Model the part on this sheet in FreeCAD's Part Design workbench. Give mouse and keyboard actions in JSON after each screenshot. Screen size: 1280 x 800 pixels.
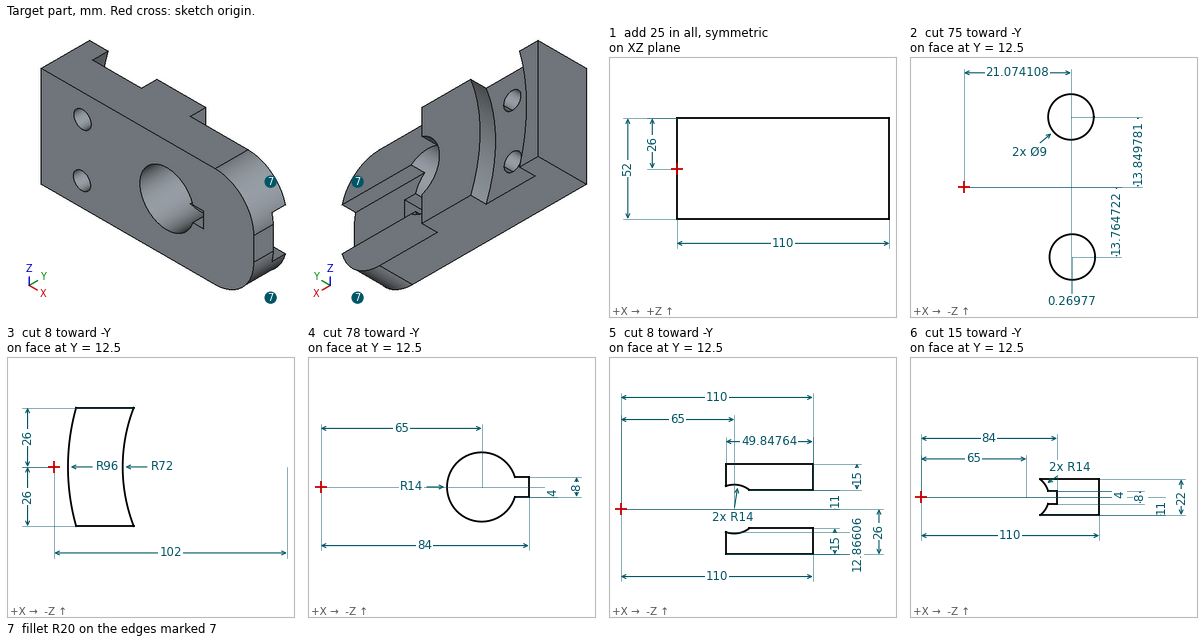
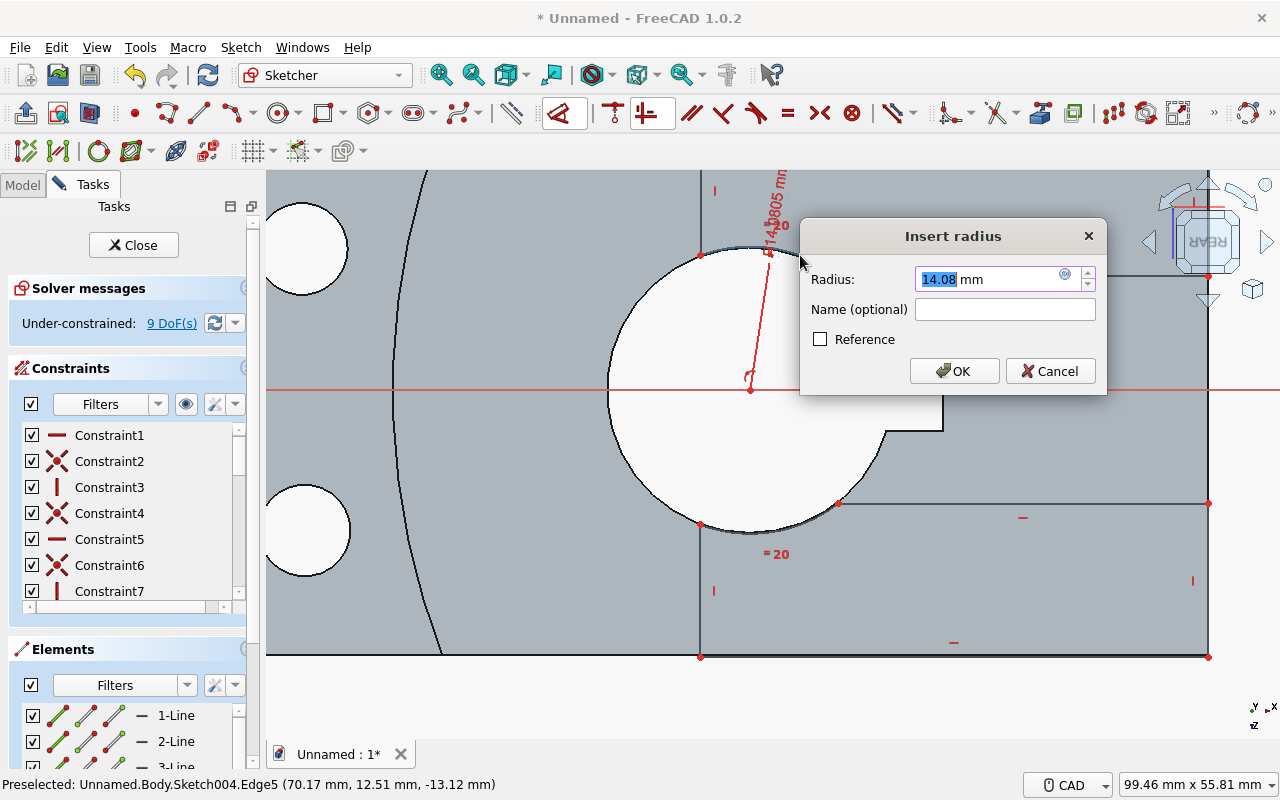
{"action": "type", "text": "14"}
{"action": "key", "text": "Return"}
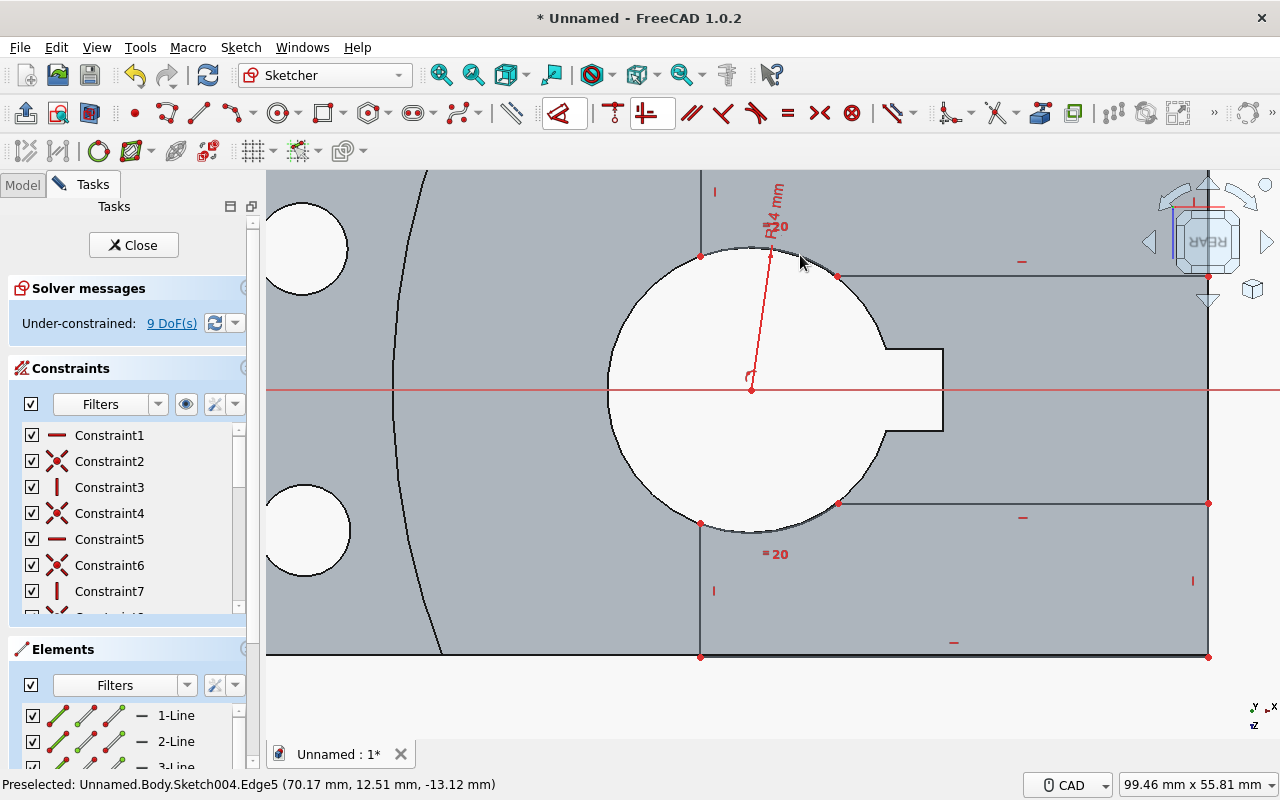
{"action": "scroll", "coordinate": [774, 533], "scroll_direction": "down", "scroll_amount": 3}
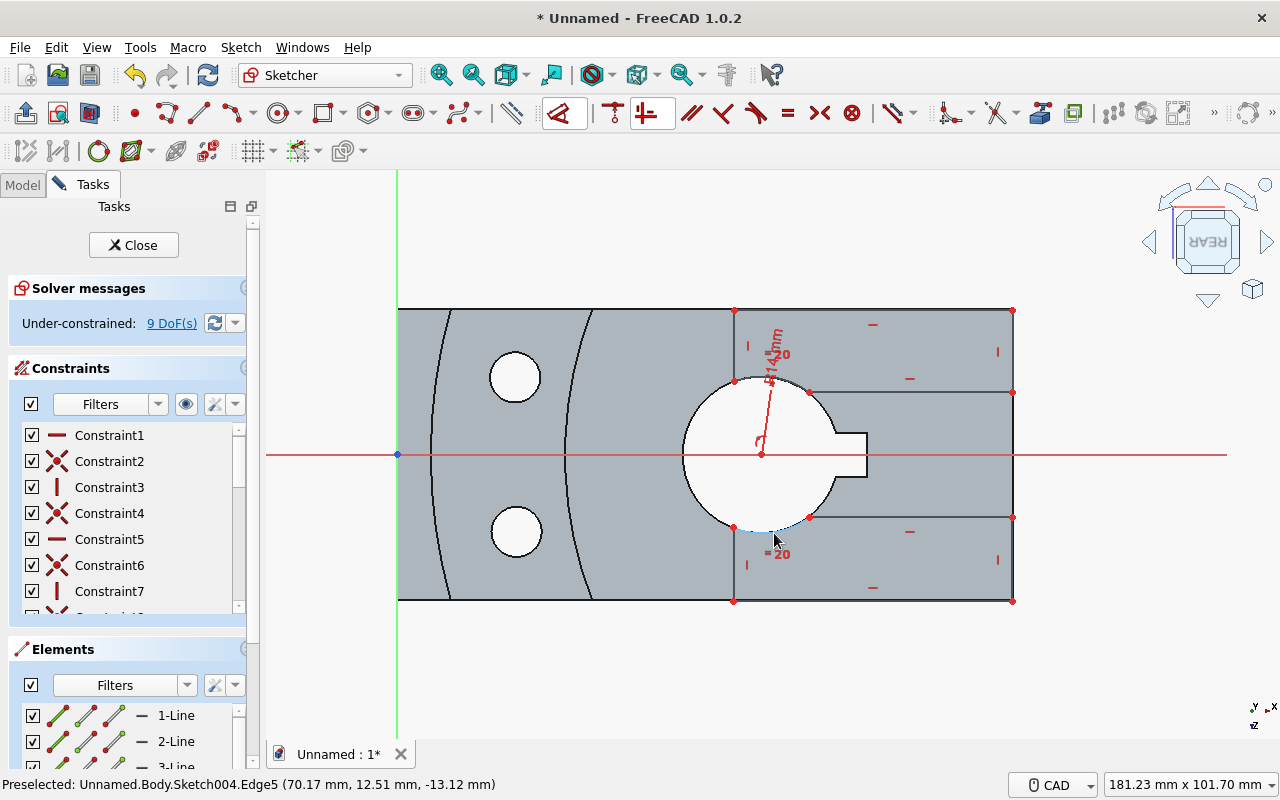
{"action": "left_click", "coordinate": [1013, 368]}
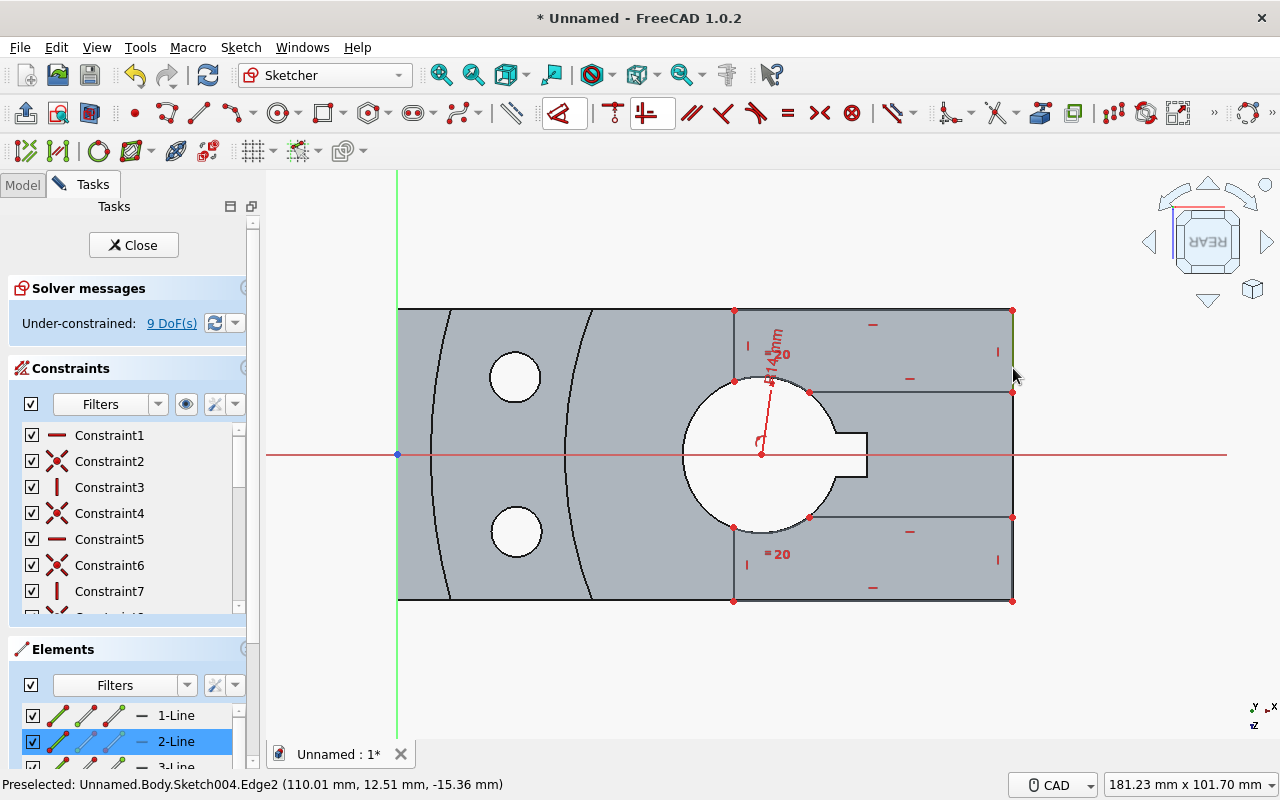
{"action": "key", "text": "i"}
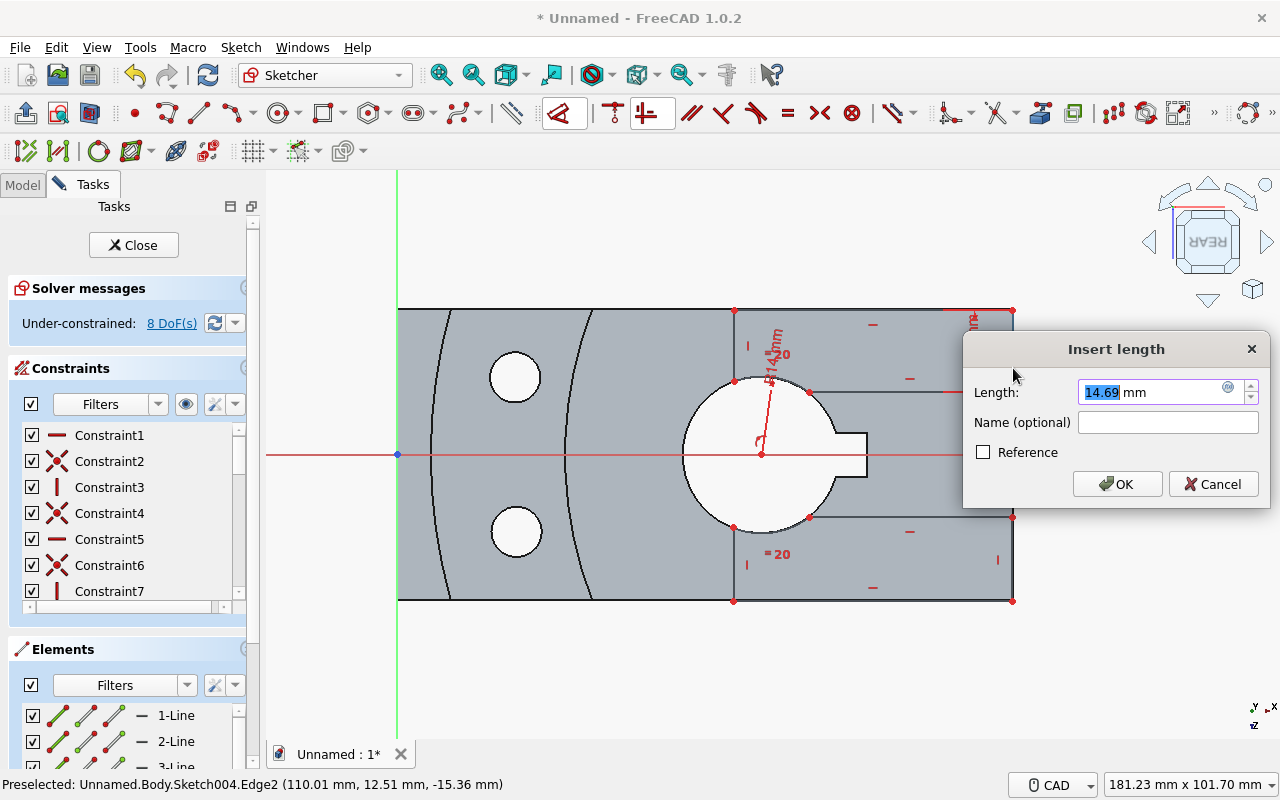
{"action": "type", "text": "15"}
{"action": "key", "text": "Return"}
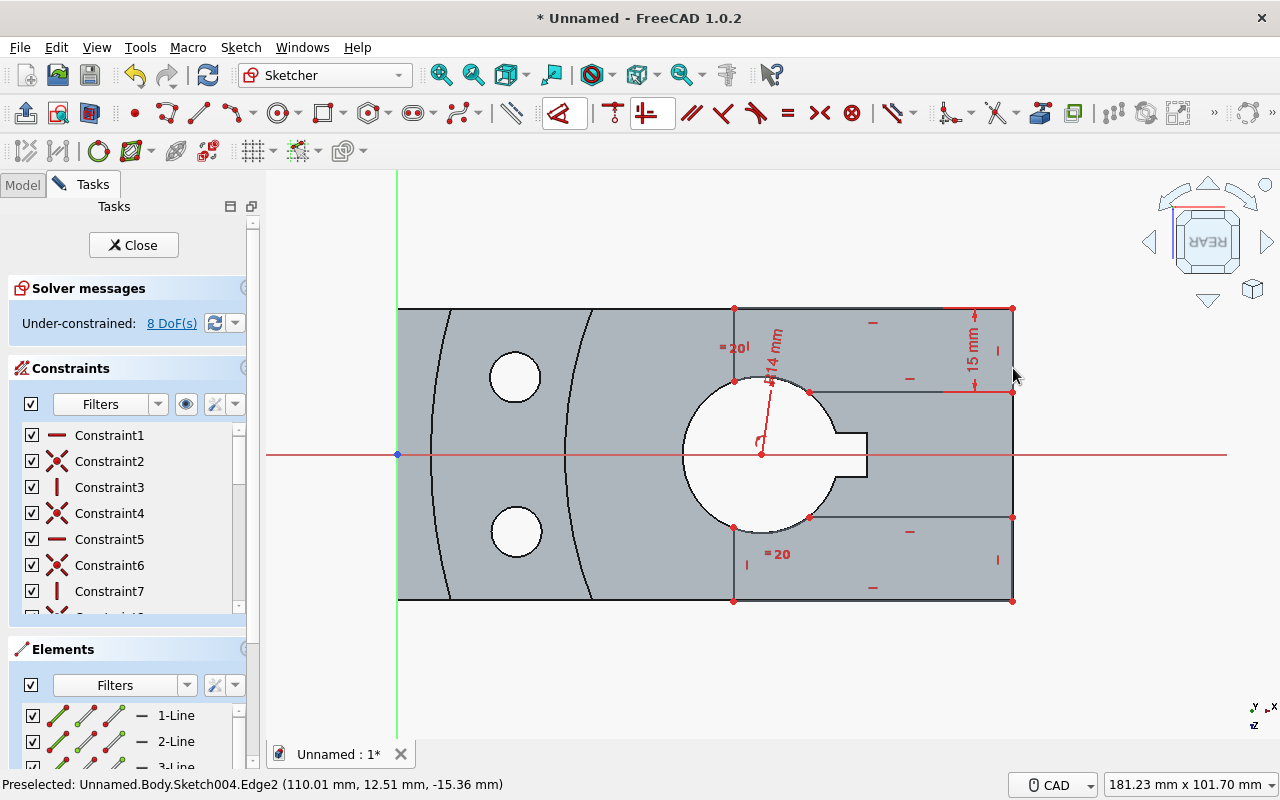
{"action": "left_click", "coordinate": [1012, 576]}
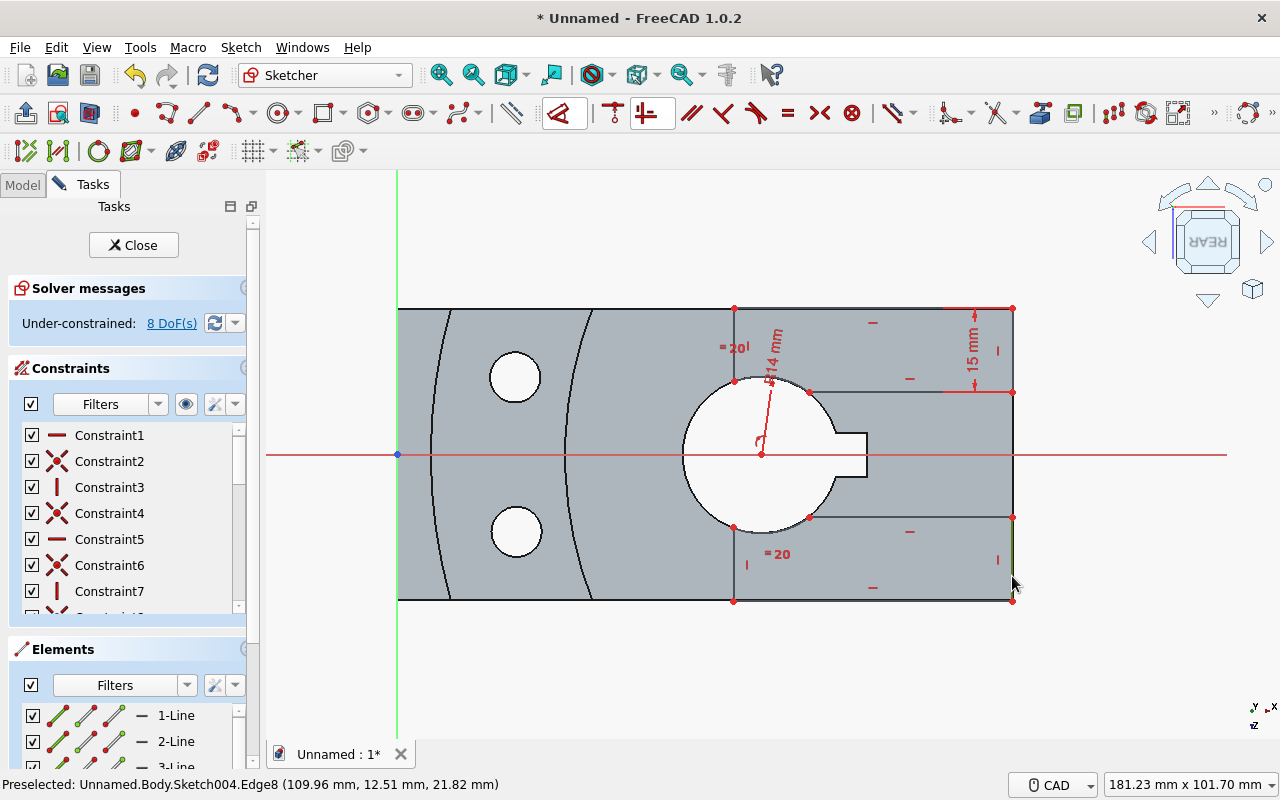
{"action": "left_click", "coordinate": [582, 114]}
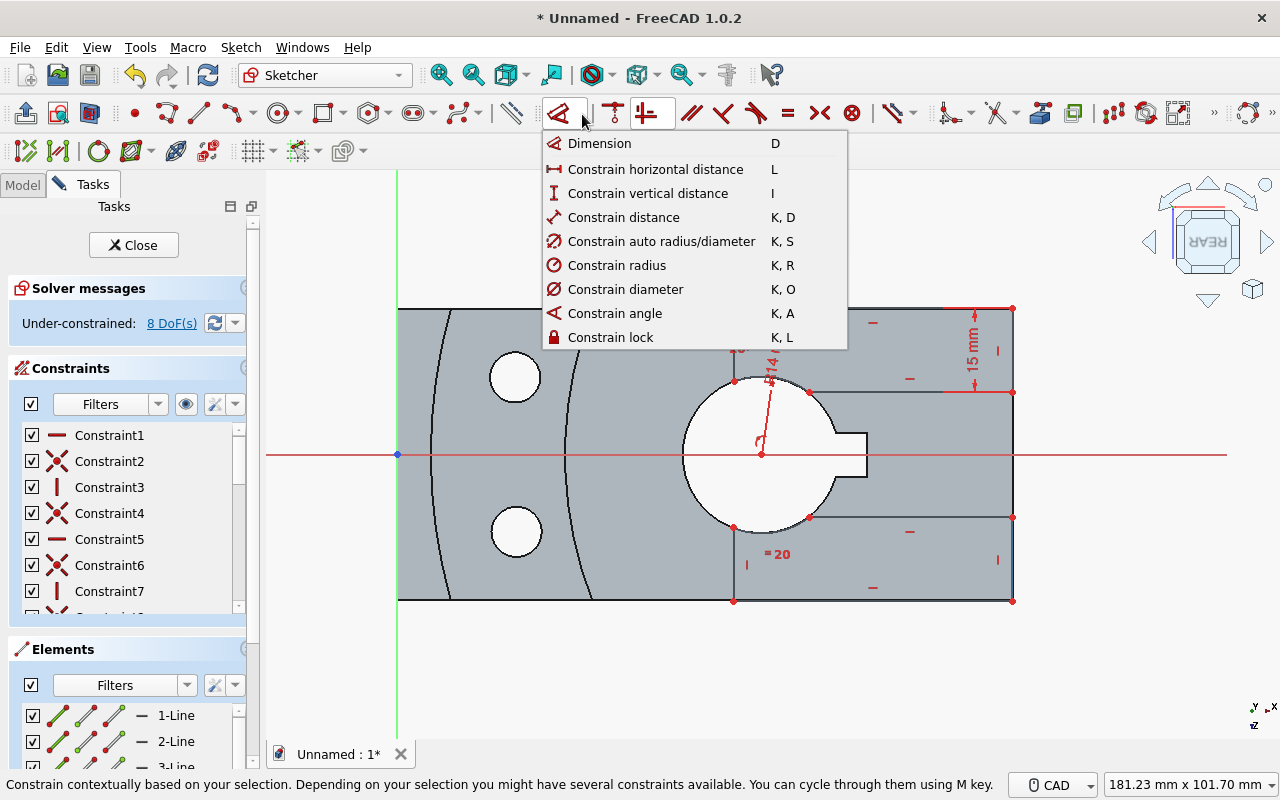
{"action": "left_click", "coordinate": [695, 193]}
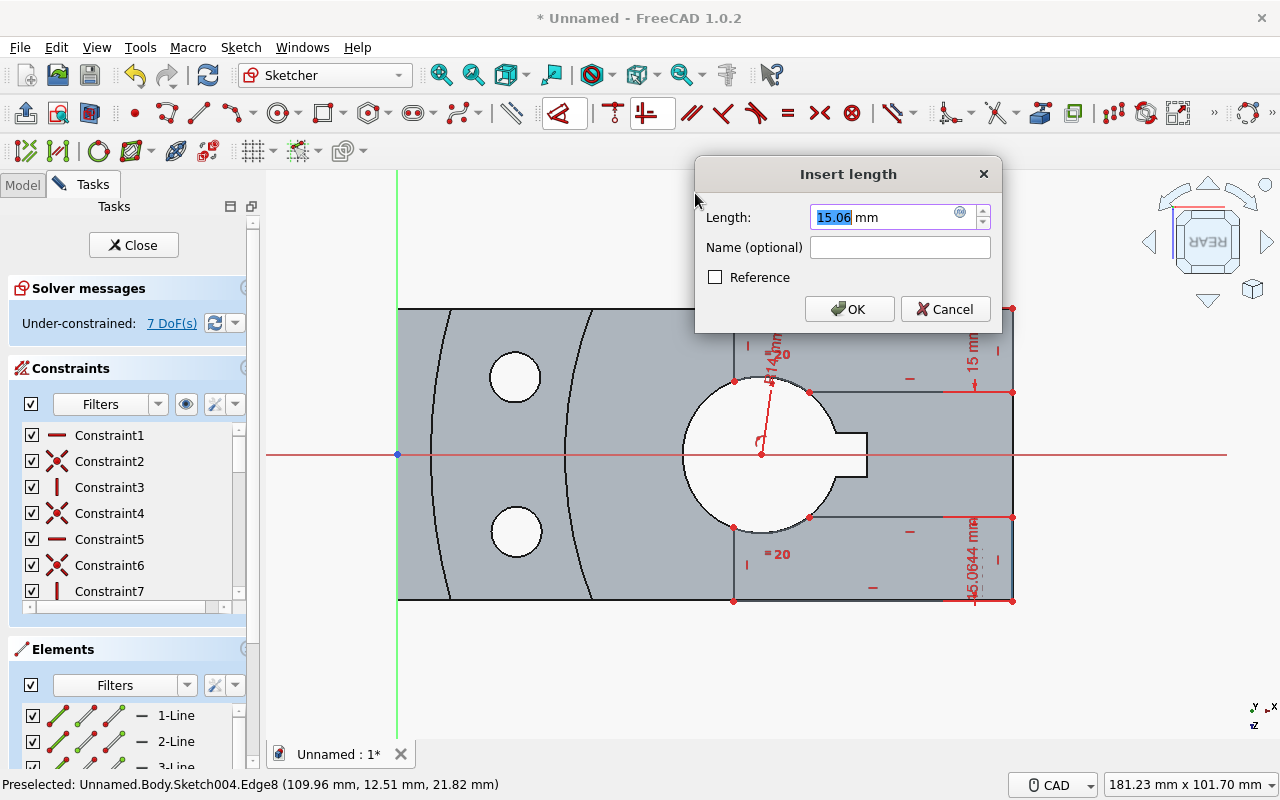
{"action": "type", "text": "15"}
{"action": "key", "text": "Return"}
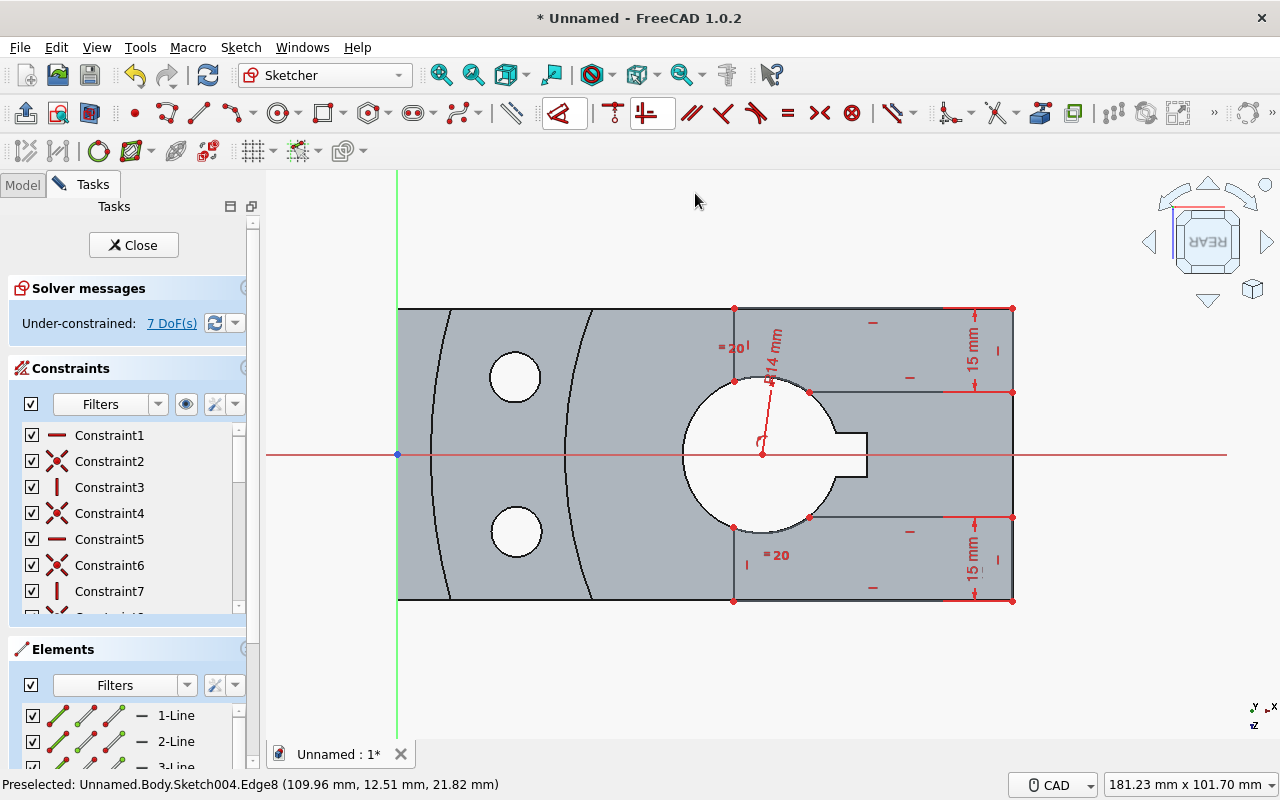
{"action": "left_click", "coordinate": [809, 392]}